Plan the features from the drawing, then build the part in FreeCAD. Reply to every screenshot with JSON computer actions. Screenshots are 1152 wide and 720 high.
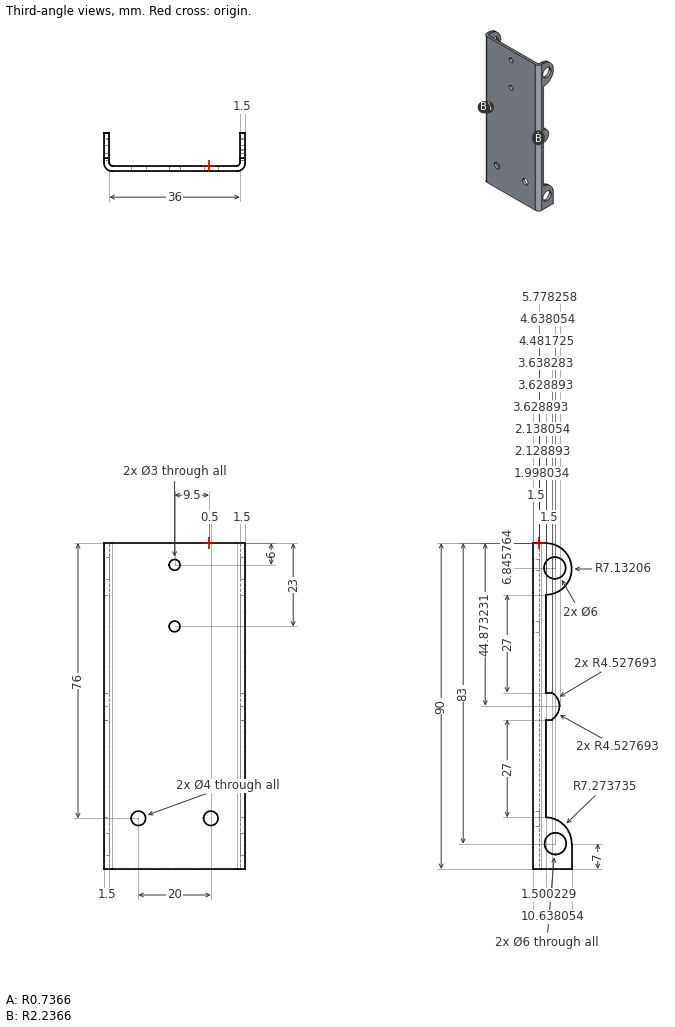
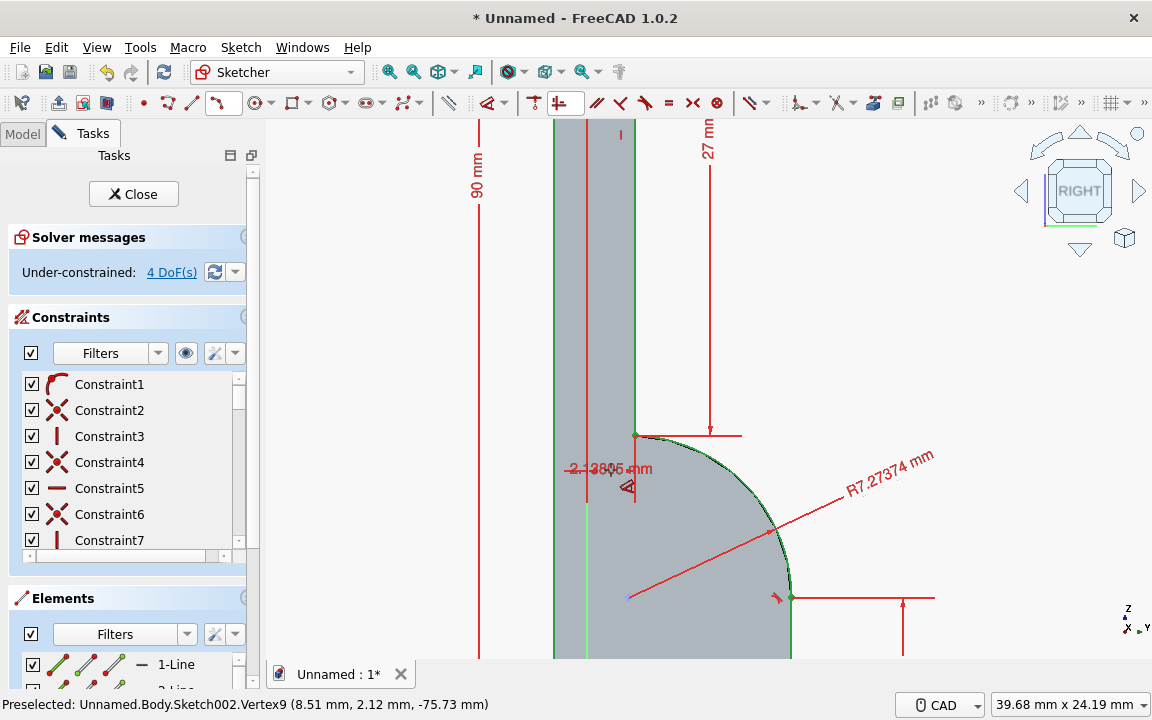
{"action": "scroll", "coordinate": [634, 516], "scroll_direction": "down", "scroll_amount": 9}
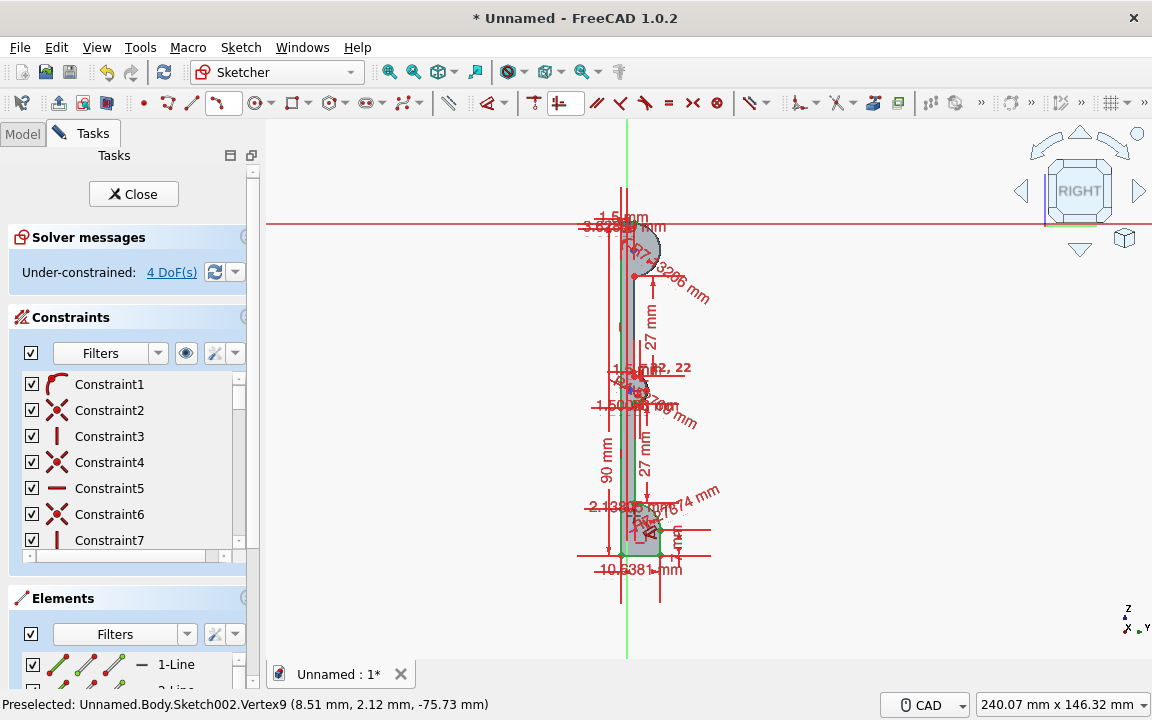
{"action": "scroll", "coordinate": [640, 376], "scroll_direction": "up", "scroll_amount": 6}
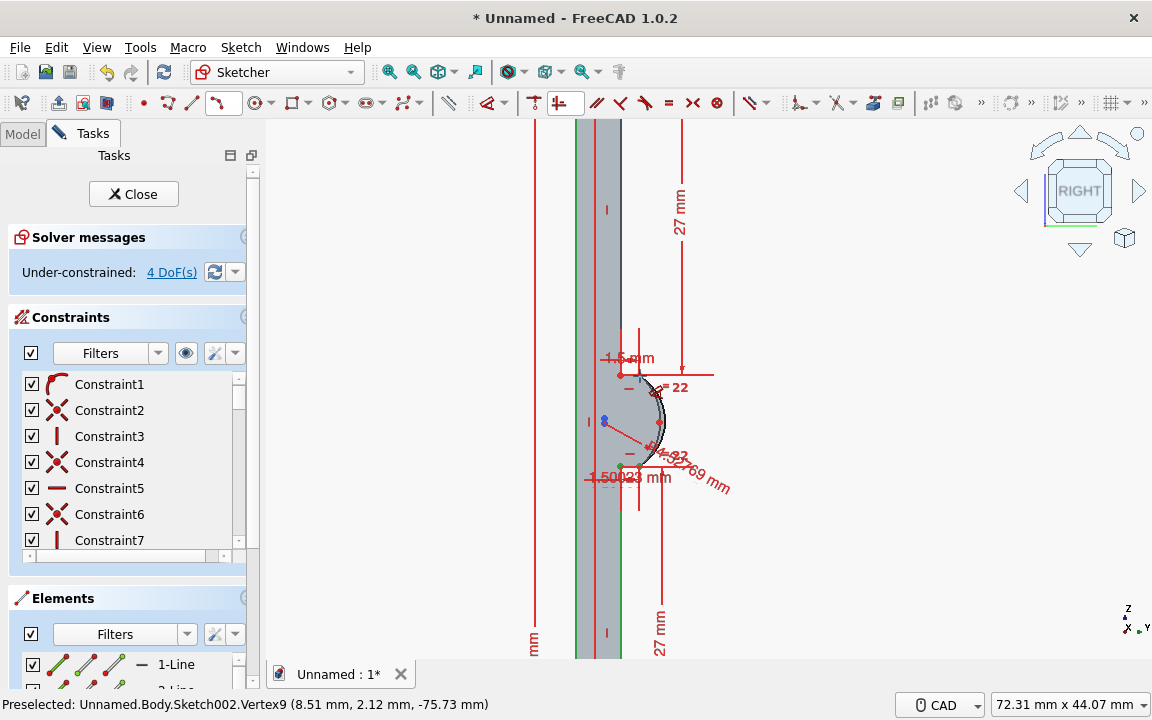
{"action": "left_click", "coordinate": [639, 375]}
{"action": "left_click", "coordinate": [617, 409]}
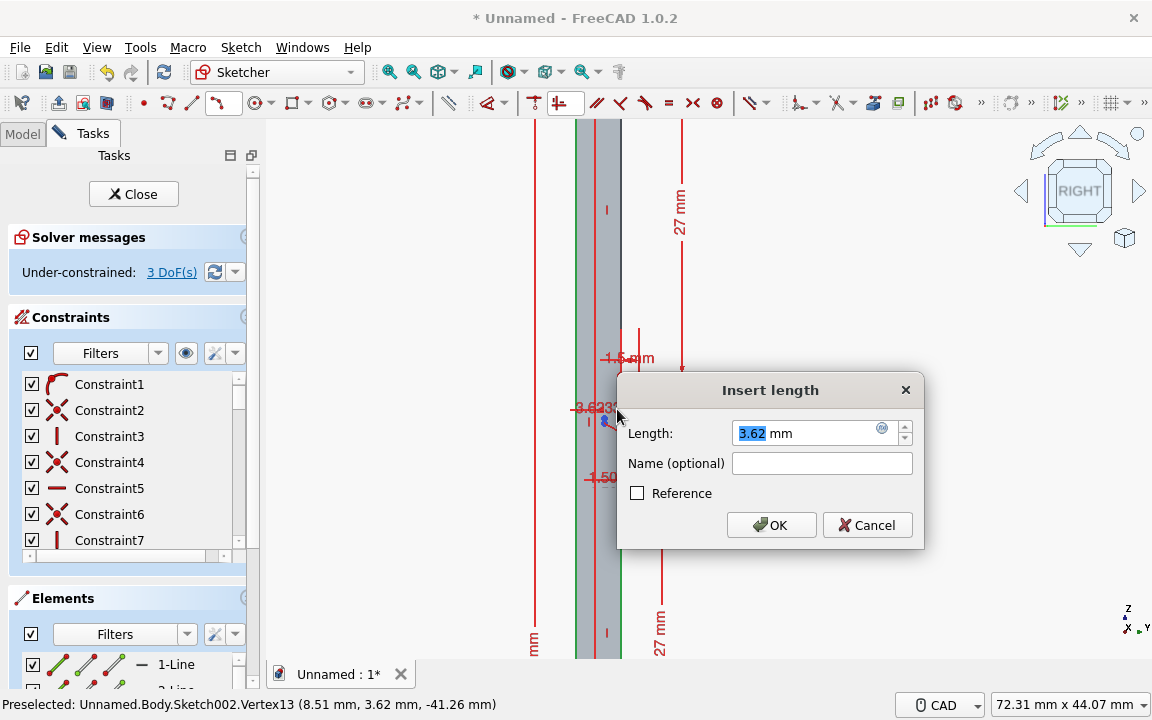
{"action": "type", "text": "3.628893"}
{"action": "key", "text": "Return"}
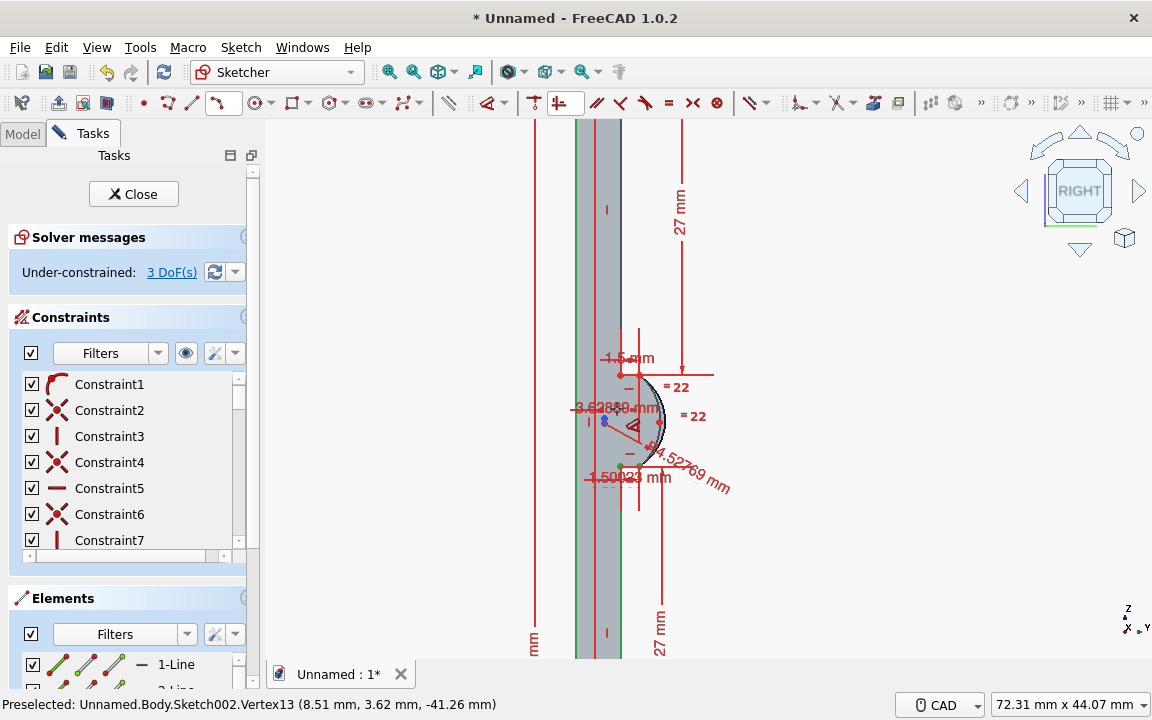
{"action": "left_click", "coordinate": [660, 422]}
{"action": "left_click", "coordinate": [612, 456]}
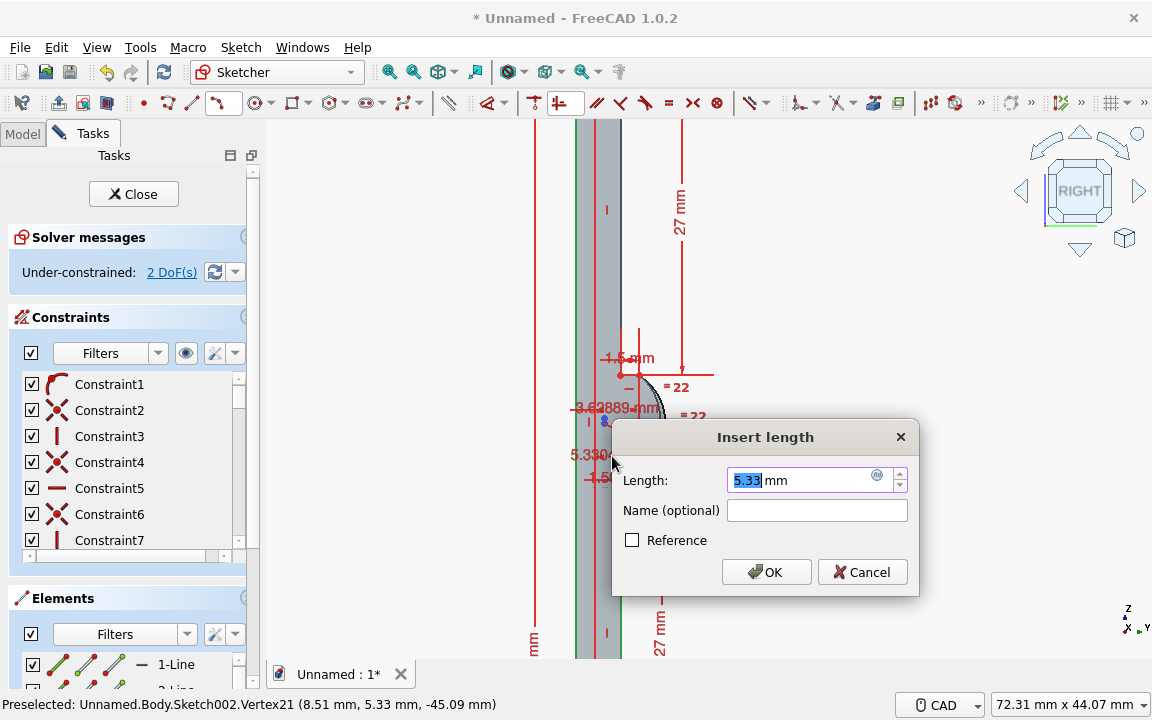
{"action": "type", "text": "5.778258"}
{"action": "key", "text": "Return"}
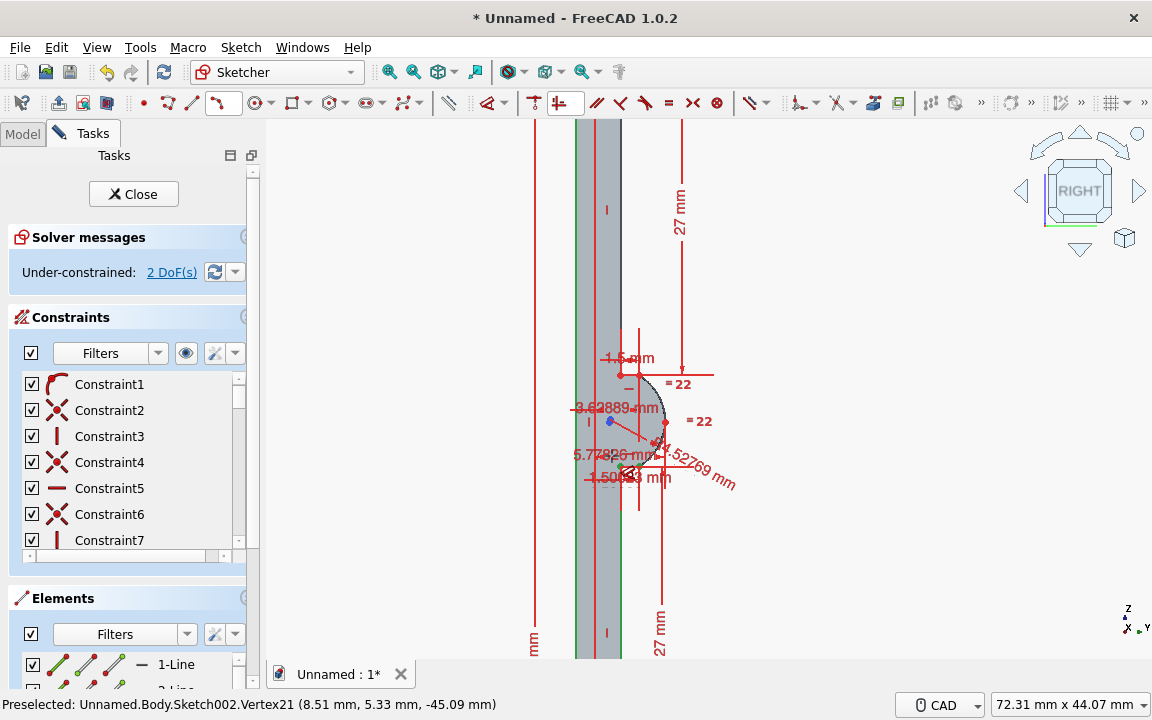
{"action": "scroll", "coordinate": [640, 375], "scroll_direction": "down", "scroll_amount": 6}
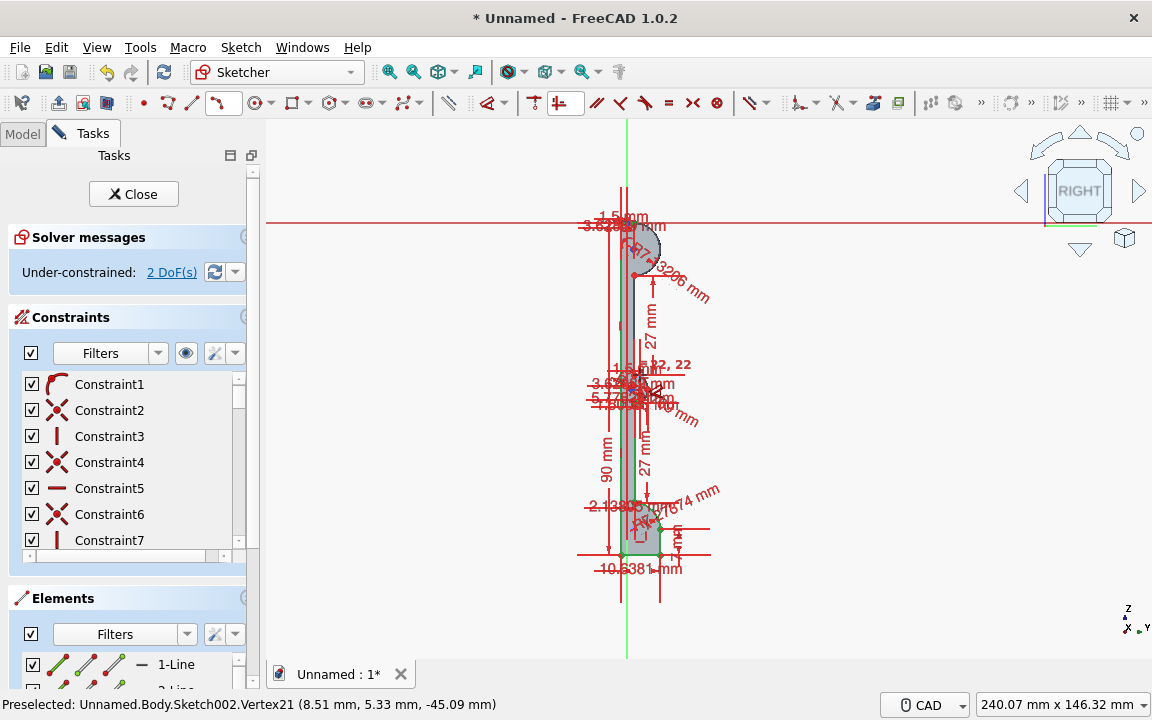
{"action": "scroll", "coordinate": [634, 249], "scroll_direction": "up", "scroll_amount": 9}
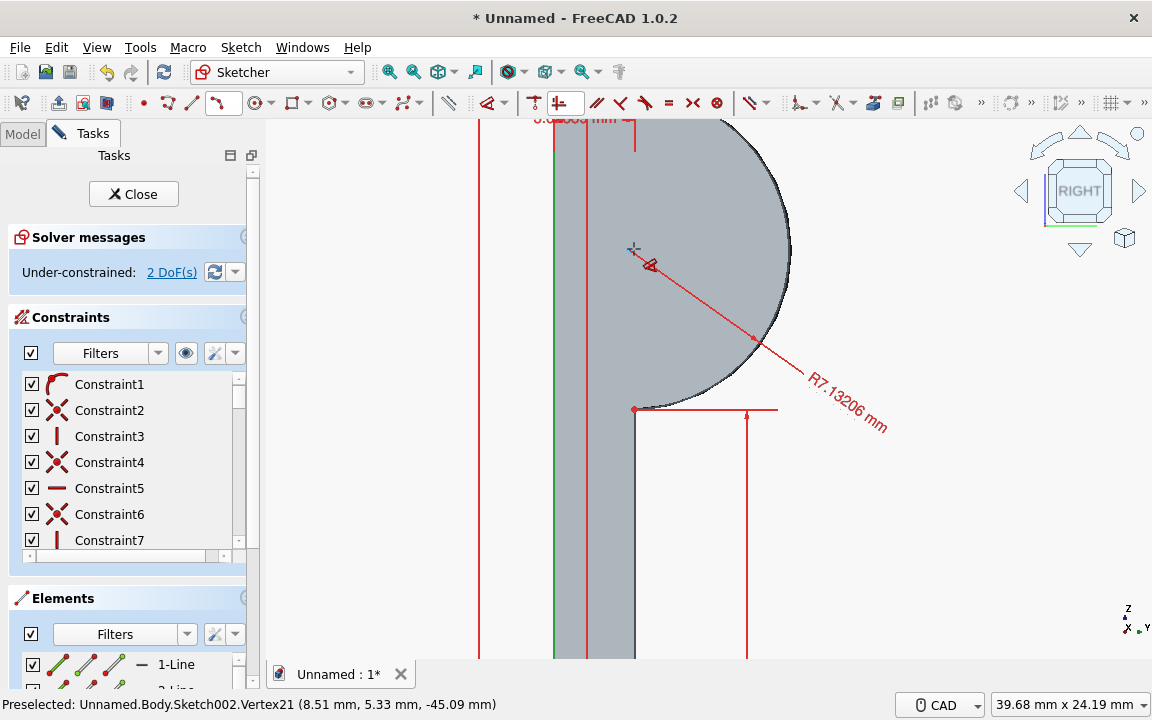
{"action": "left_click", "coordinate": [630, 250]}
{"action": "left_click", "coordinate": [609, 284]}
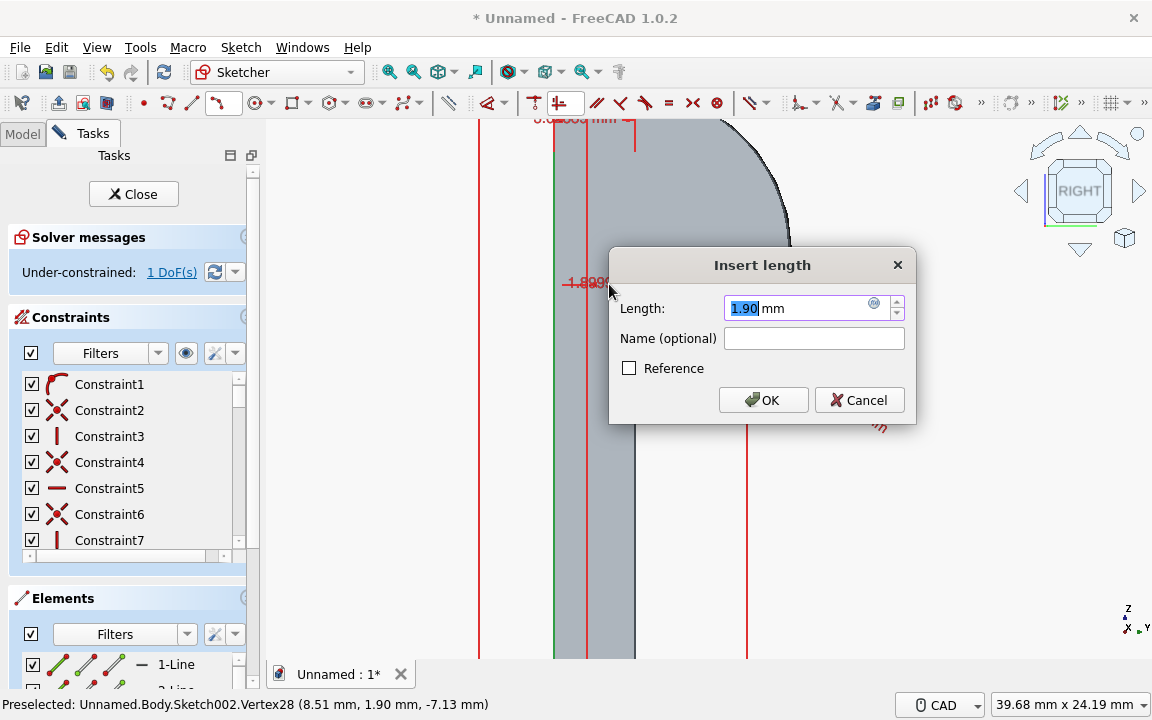
{"action": "type", "text": "1.998034"}
{"action": "key", "text": "Return"}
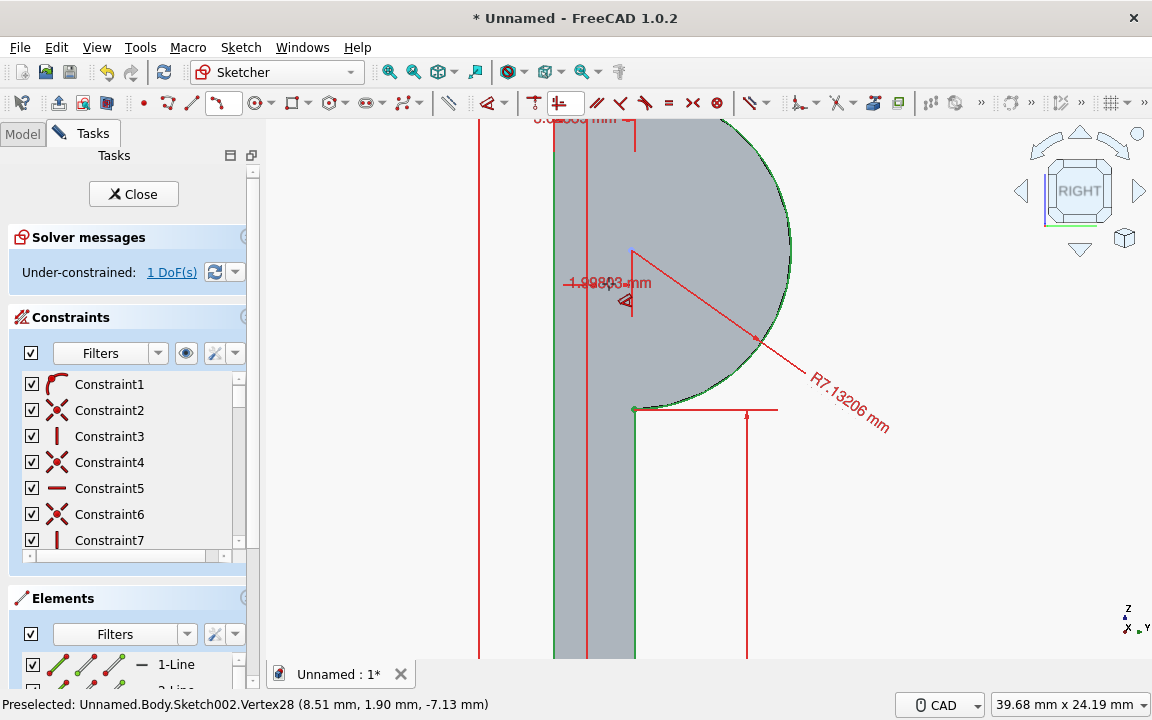
{"action": "scroll", "coordinate": [634, 249], "scroll_direction": "down", "scroll_amount": 9}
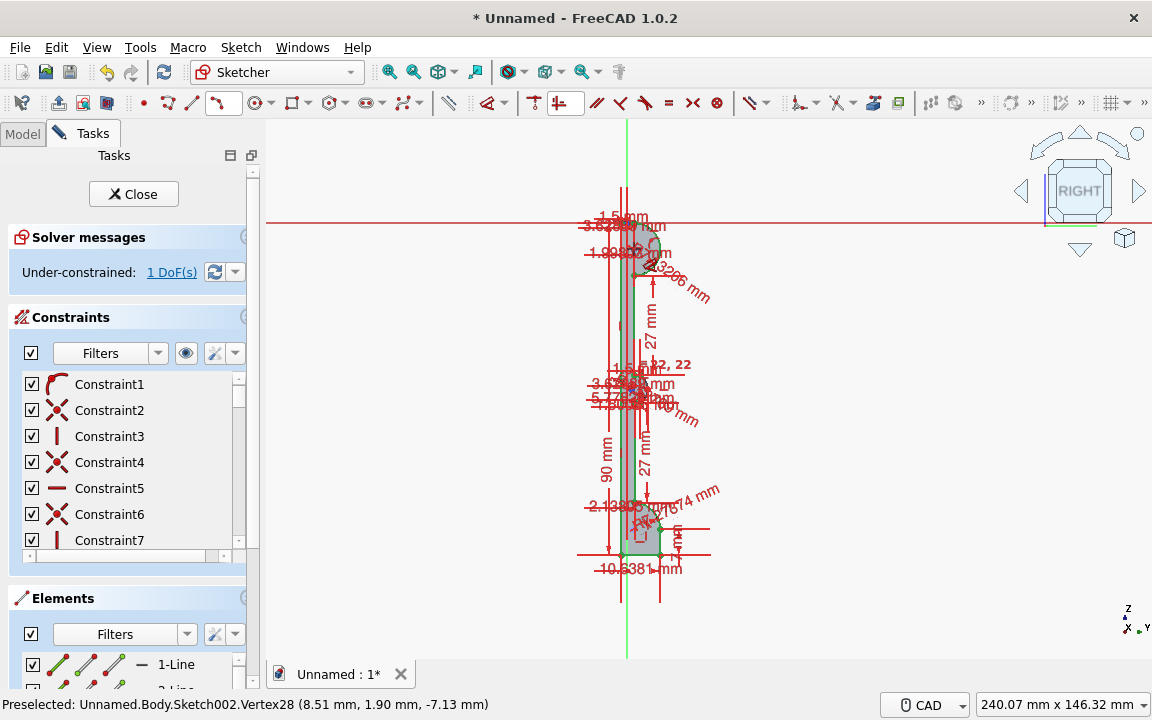
{"action": "left_click", "coordinate": [648, 390]}
{"action": "left_click", "coordinate": [593, 306]}